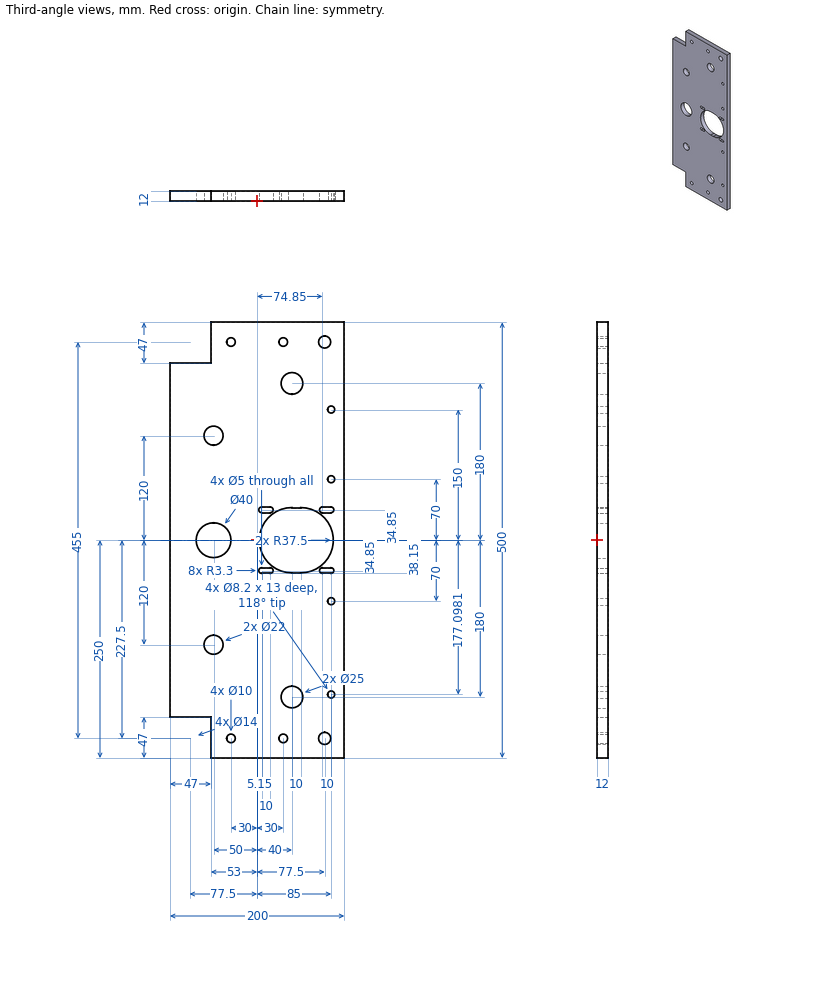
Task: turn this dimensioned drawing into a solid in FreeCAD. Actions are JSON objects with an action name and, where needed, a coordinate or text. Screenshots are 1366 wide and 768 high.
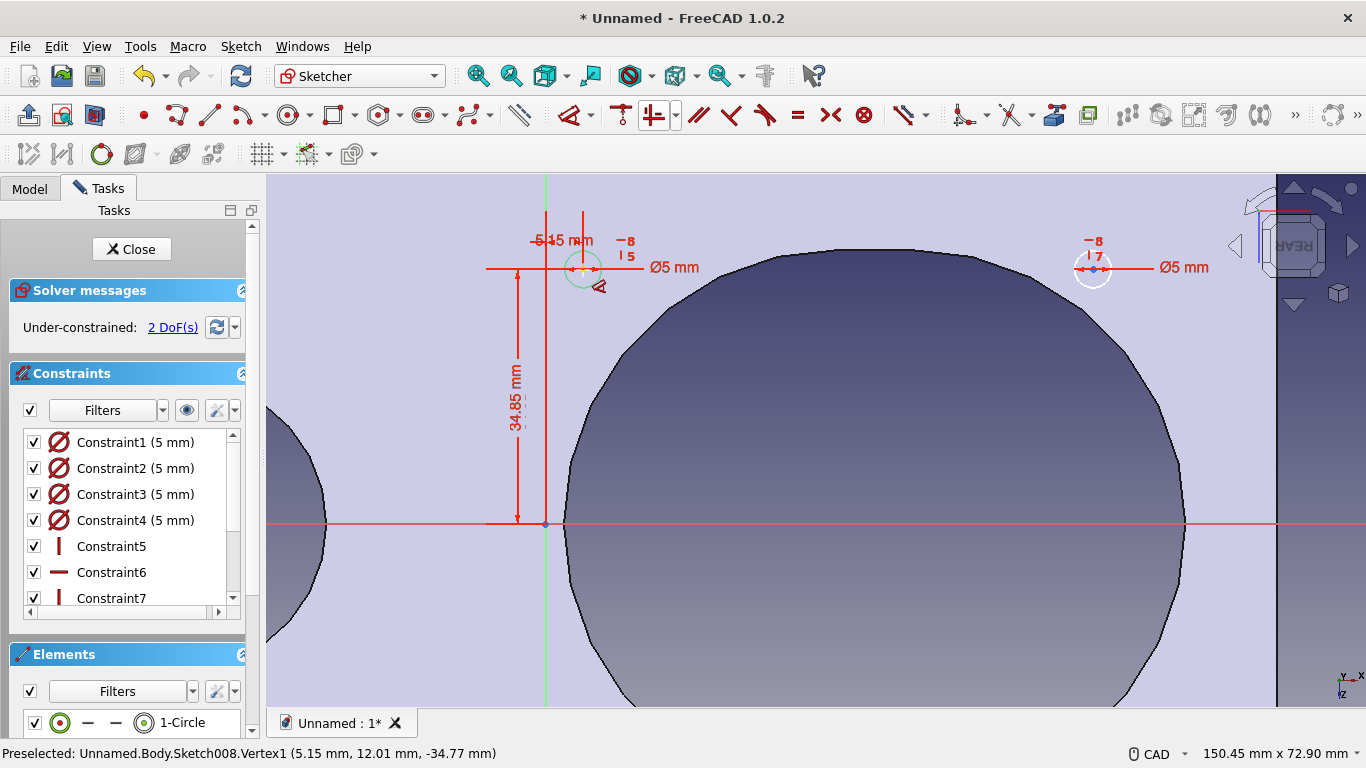
{"action": "left_click", "coordinate": [583, 612]}
{"action": "left_click", "coordinate": [524, 526]}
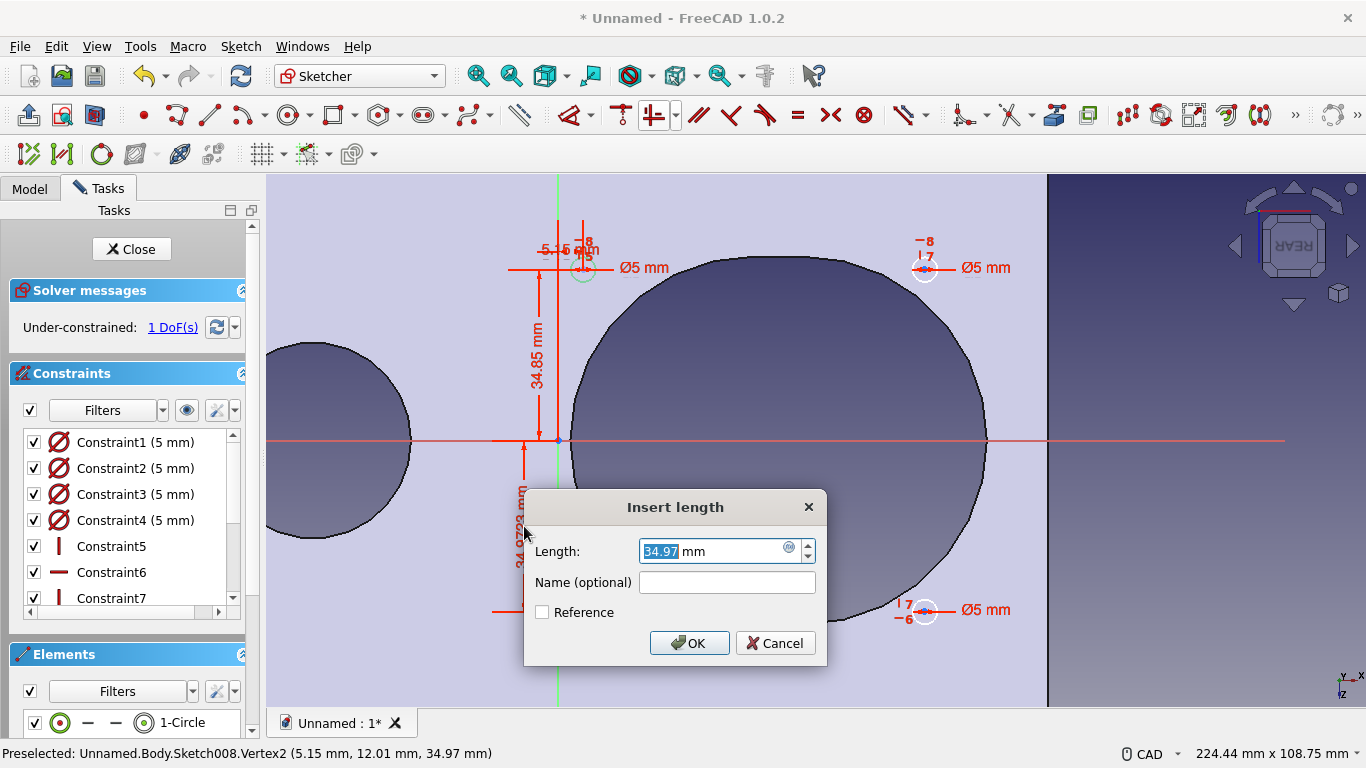
{"action": "type", "text": "34.85"}
{"action": "key", "text": "Return"}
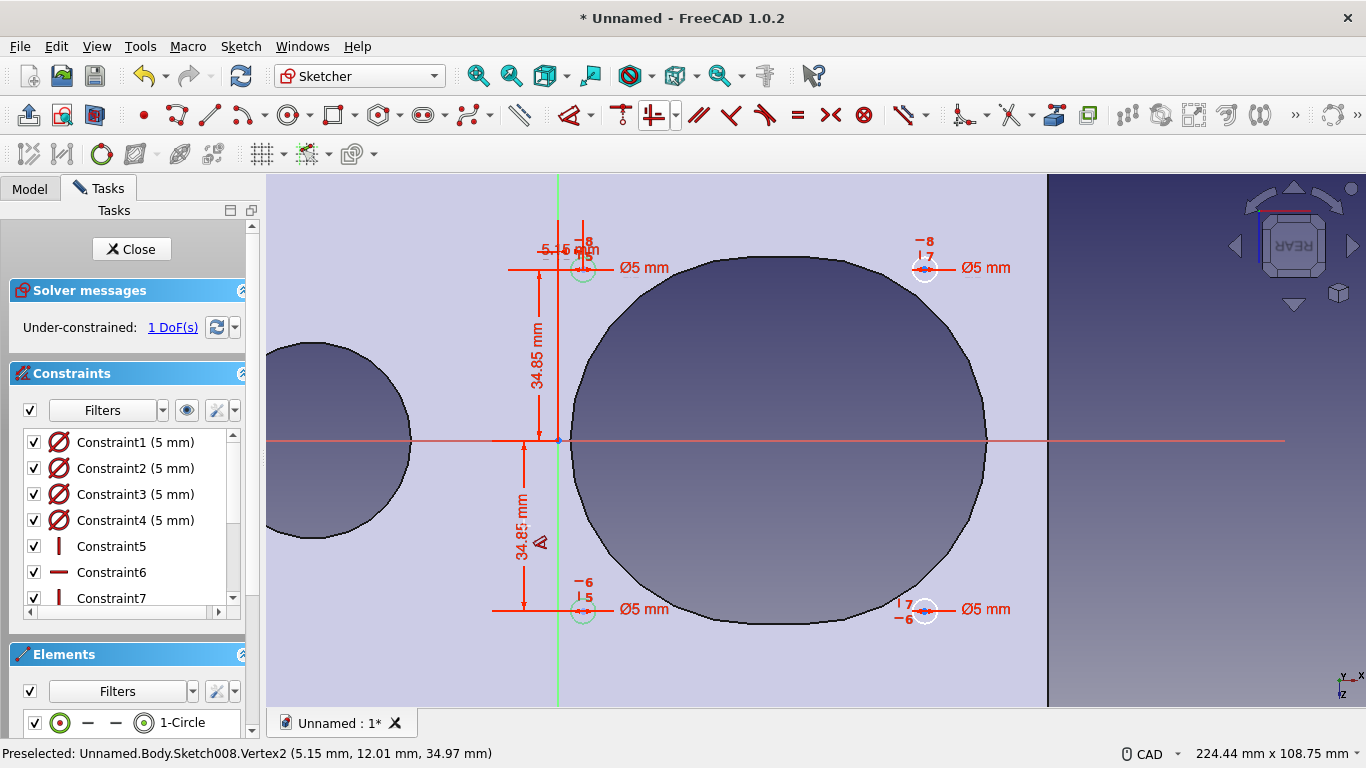
{"action": "left_click", "coordinate": [925, 611]}
{"action": "left_click", "coordinate": [742, 645]}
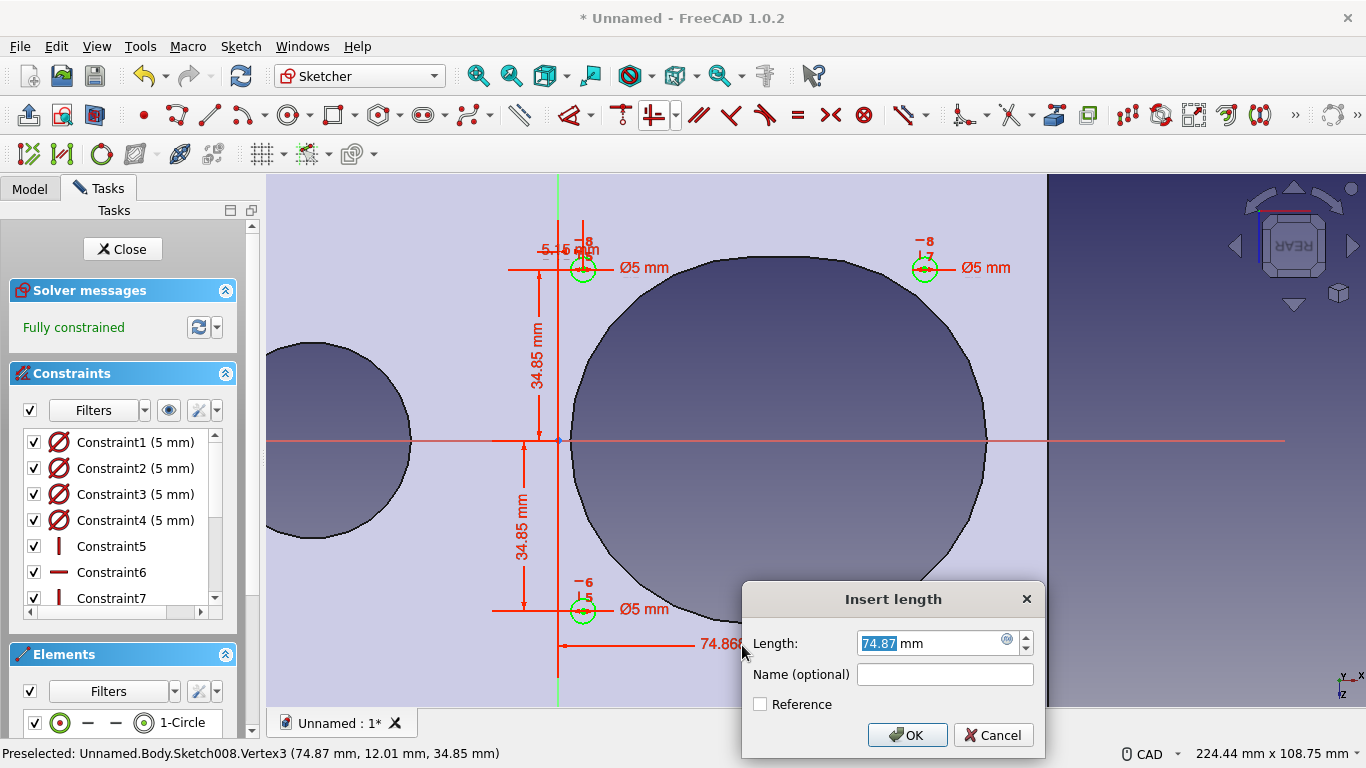
{"action": "type", "text": "74.85"}
{"action": "key", "text": "Return"}
{"action": "key", "text": "Escape"}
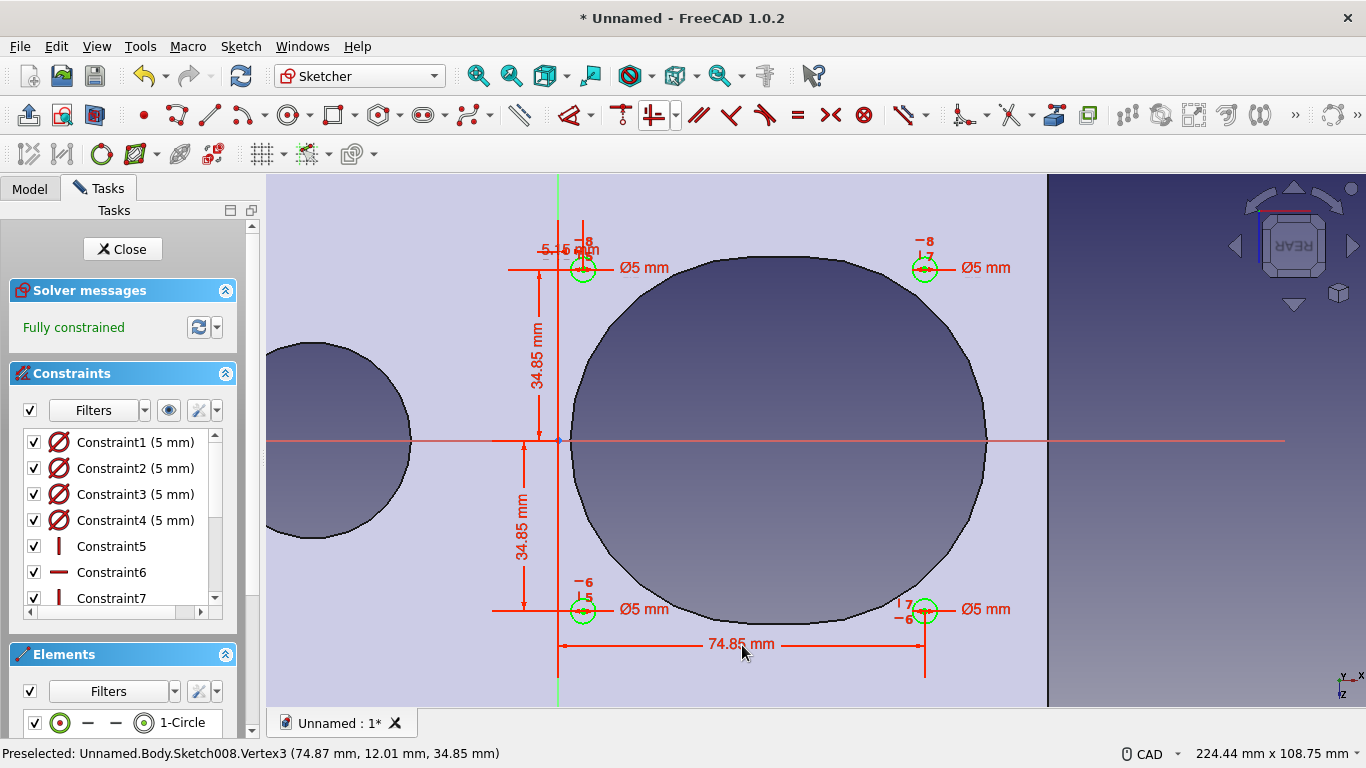
{"action": "left_click", "coordinate": [123, 249]}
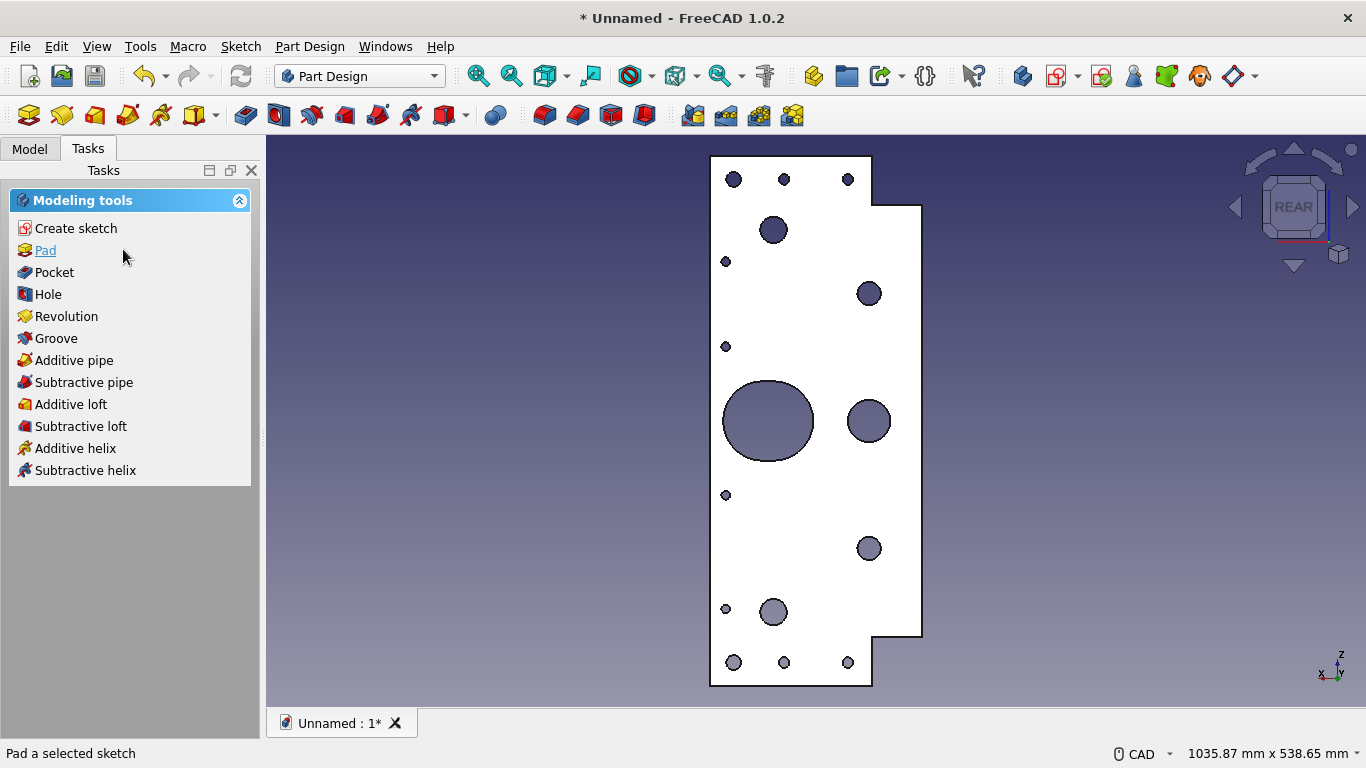
{"action": "left_click", "coordinate": [279, 116]}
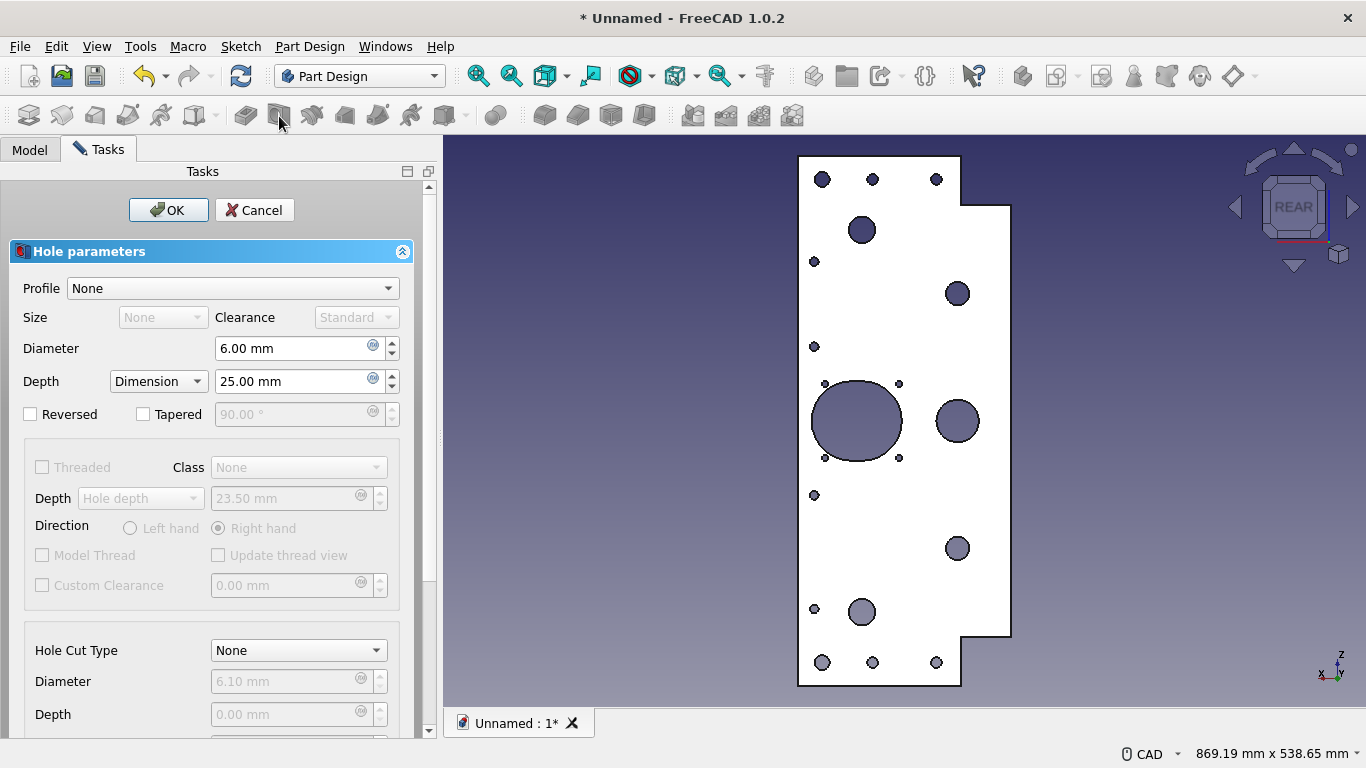
{"action": "triple_click", "coordinate": [300, 348]}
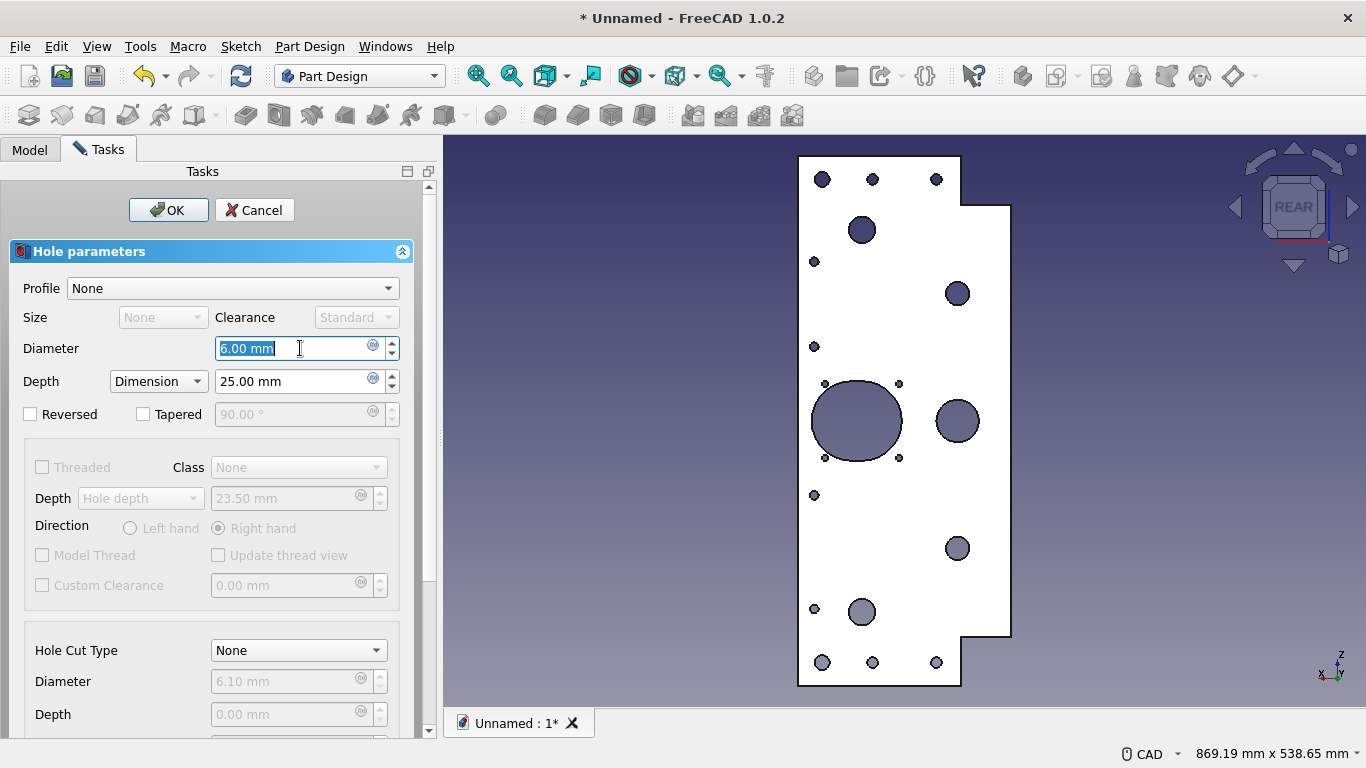
{"action": "type", "text": "5"}
{"action": "key", "text": "Tab"}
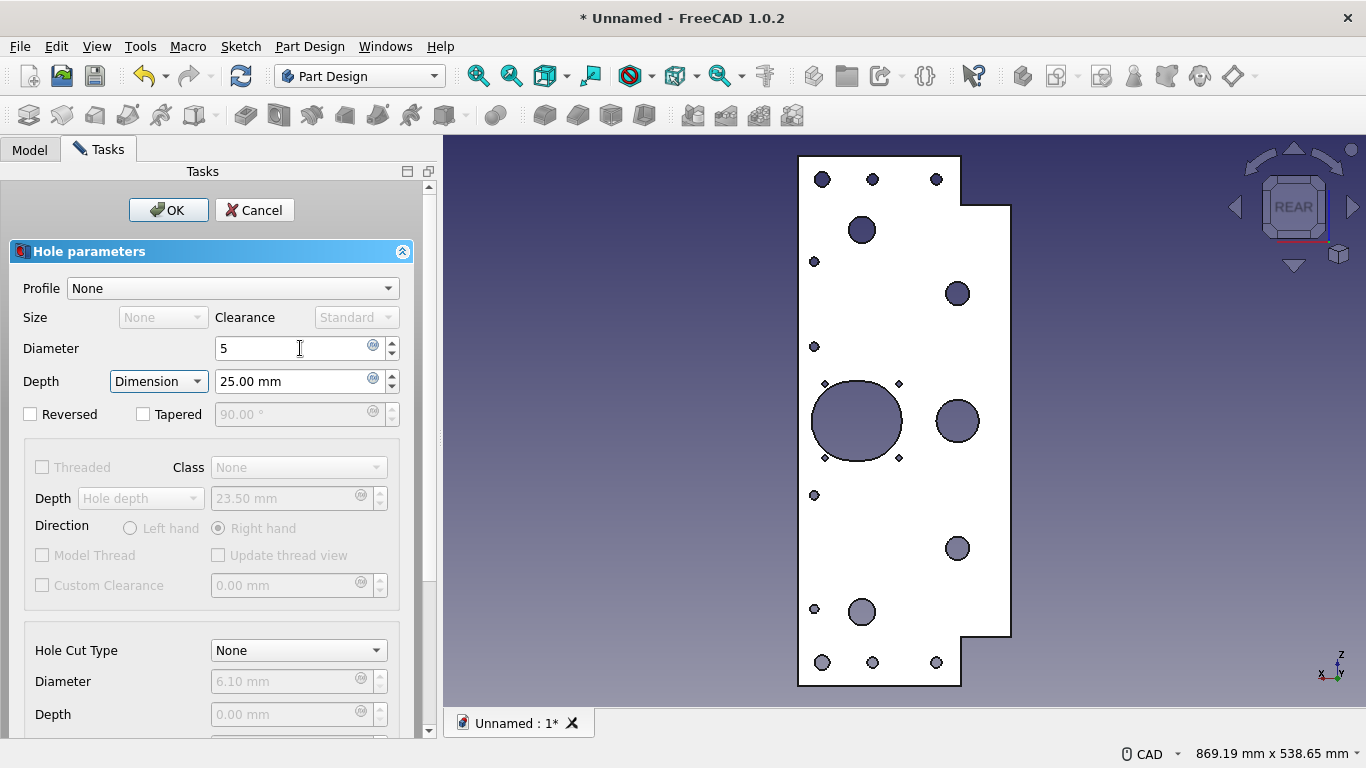
{"action": "left_click", "coordinate": [160, 382]}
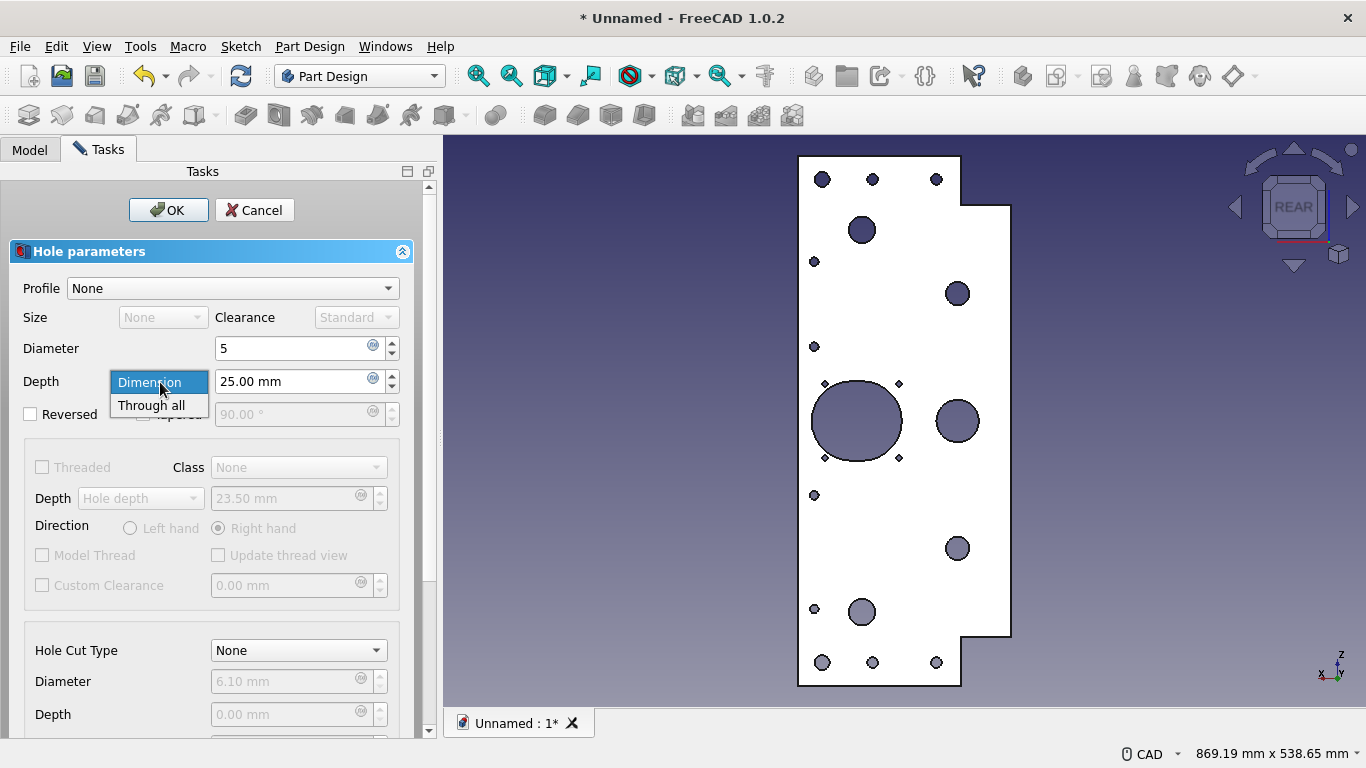
{"action": "left_click", "coordinate": [158, 406]}